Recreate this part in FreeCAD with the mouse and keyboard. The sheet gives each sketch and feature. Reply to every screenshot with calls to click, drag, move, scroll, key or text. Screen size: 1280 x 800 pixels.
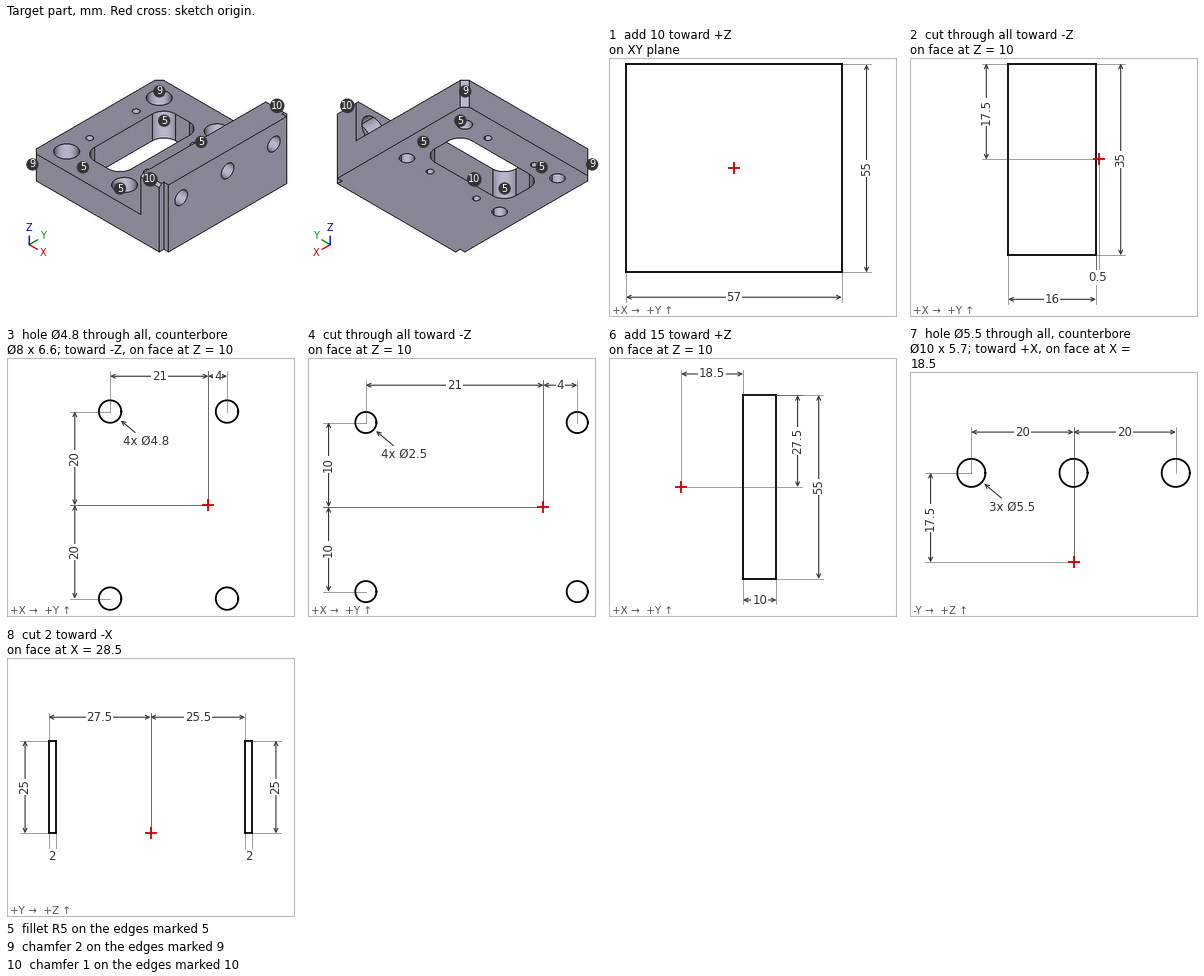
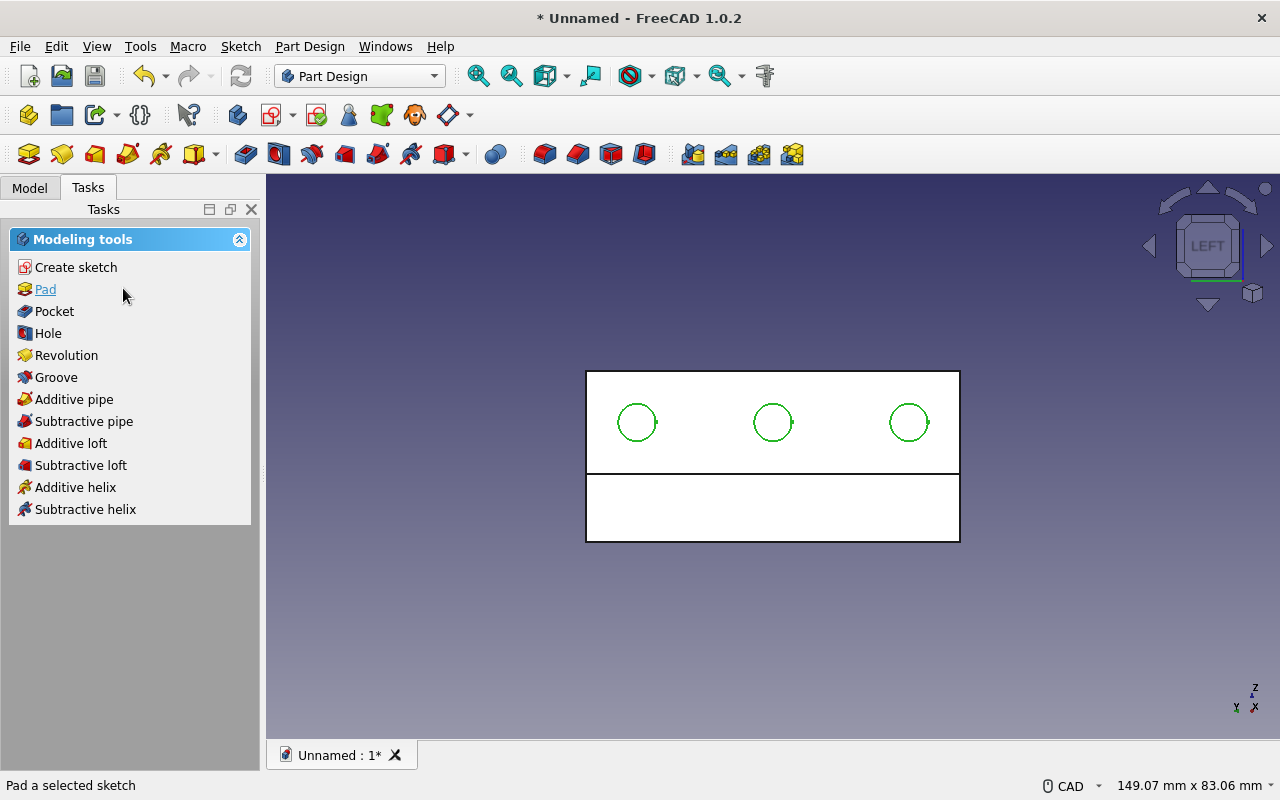
click(279, 154)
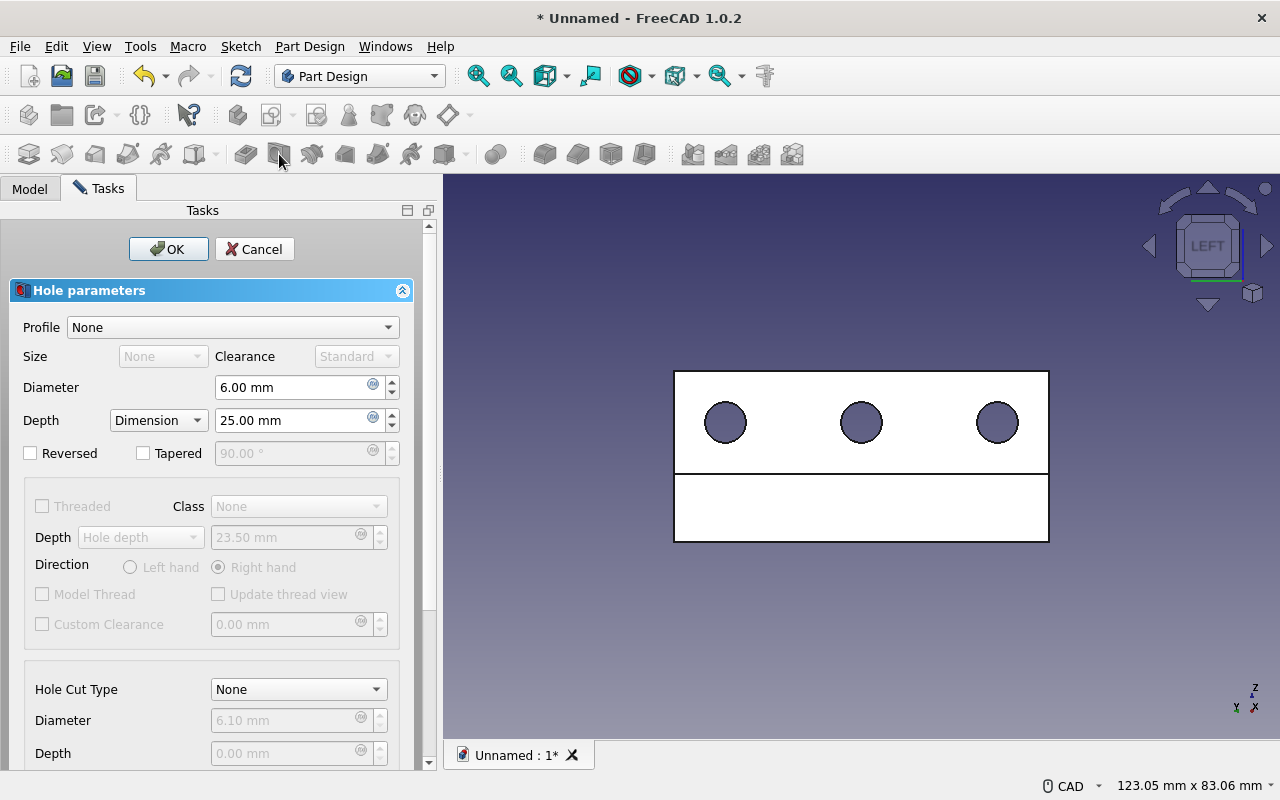
triple_click(300, 388)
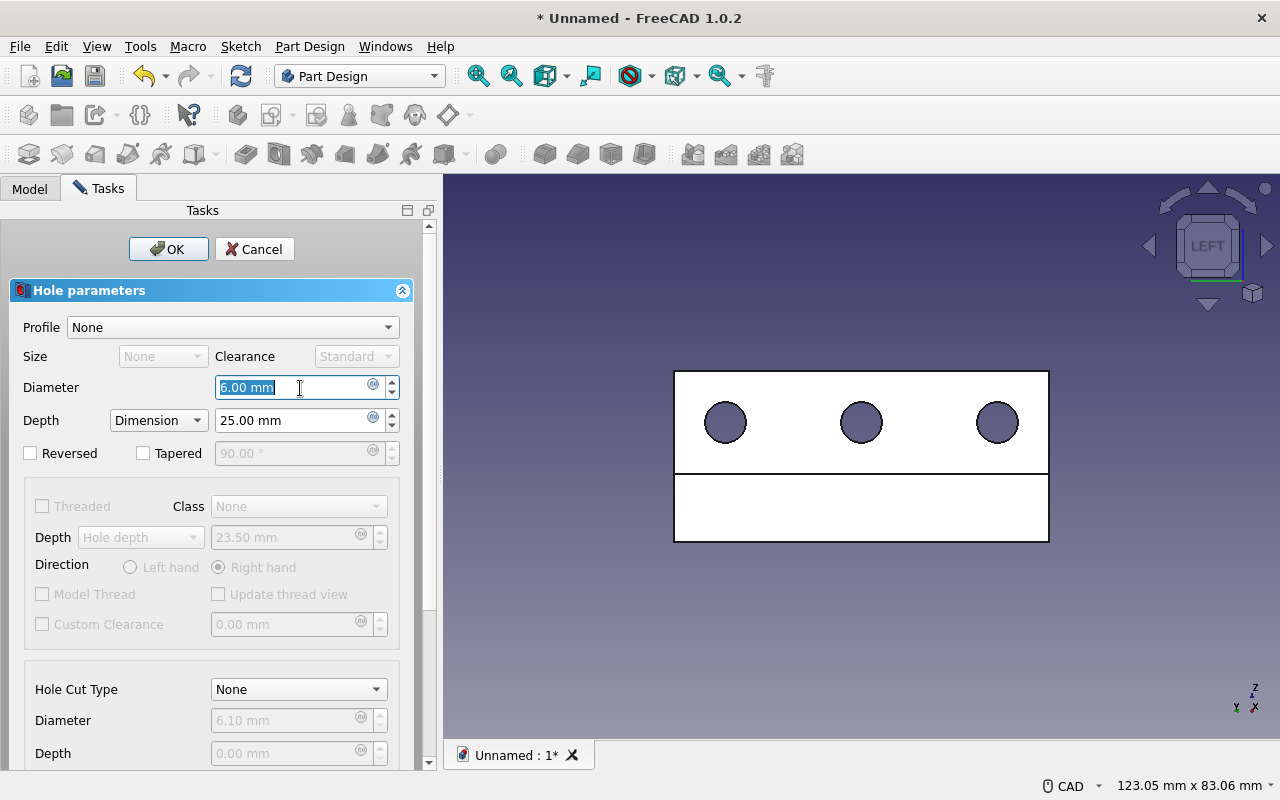
text(5.5)
key(Tab)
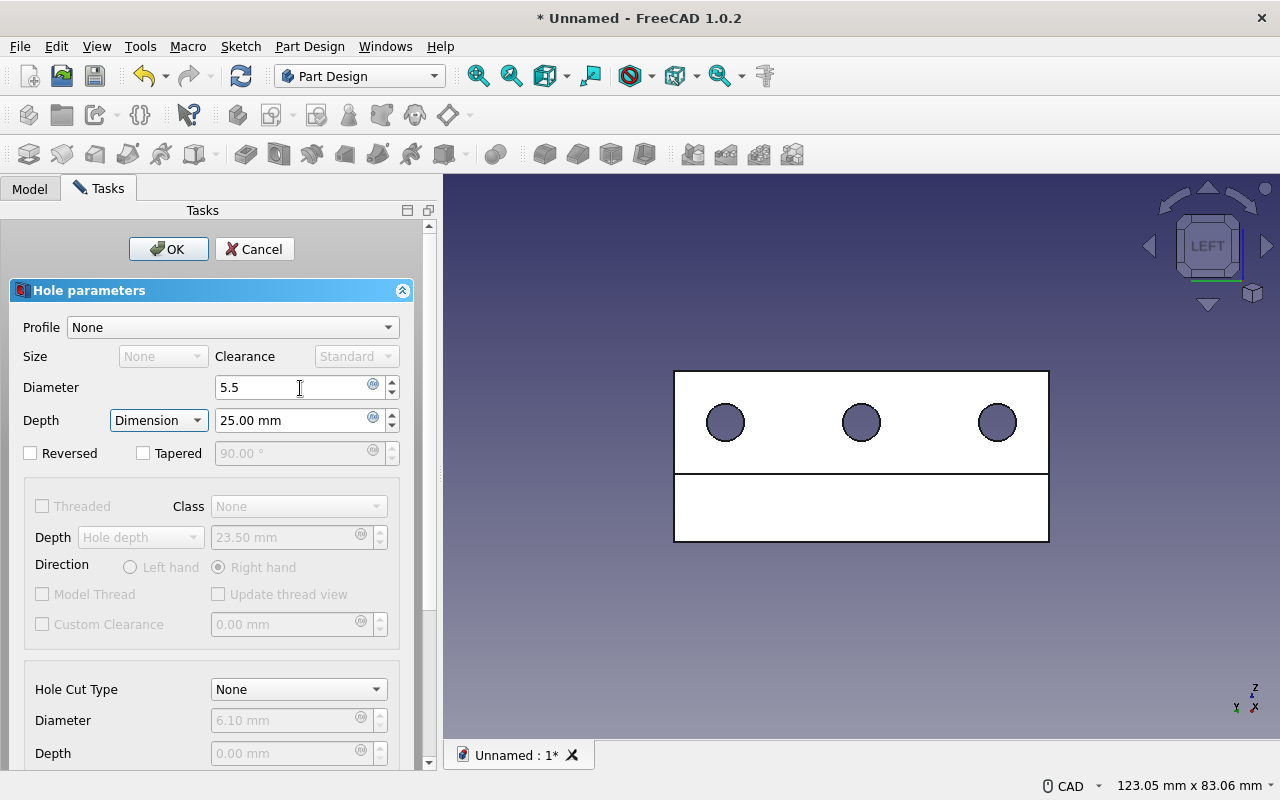
click(160, 420)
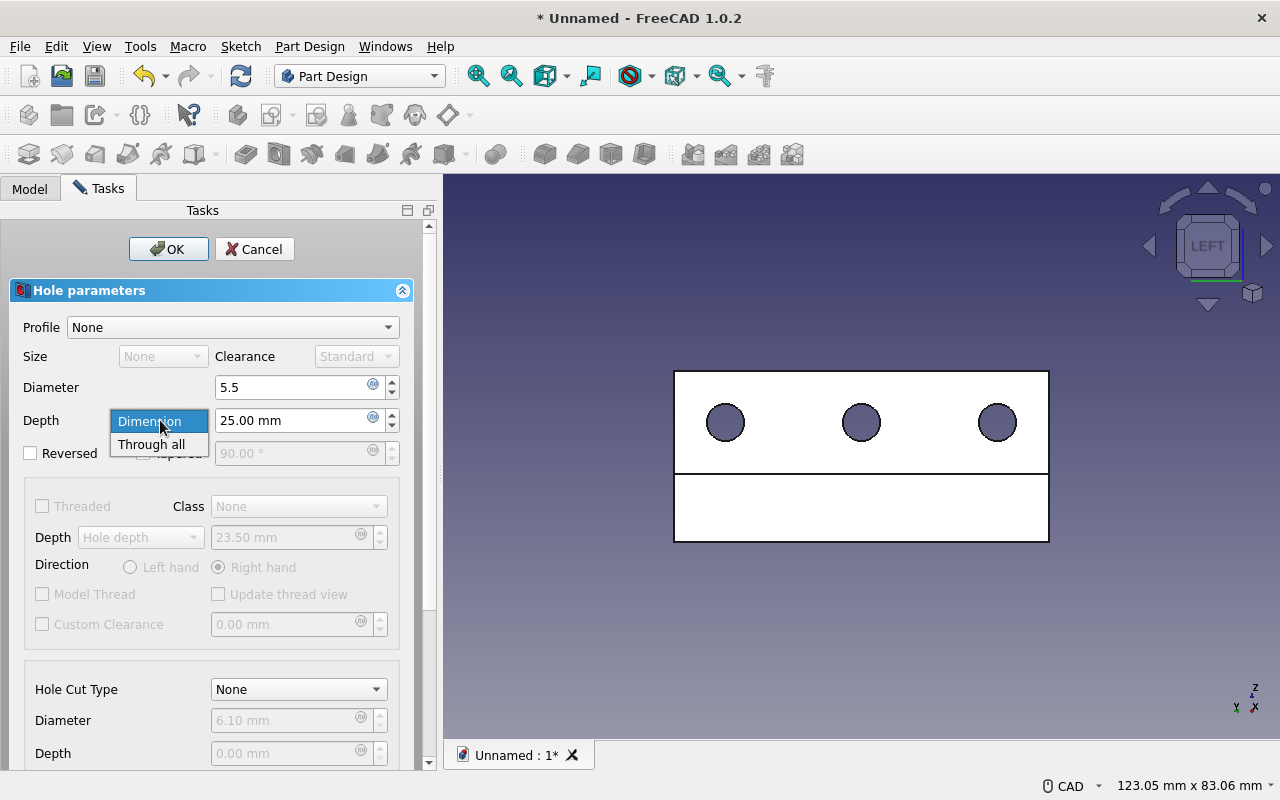
click(158, 444)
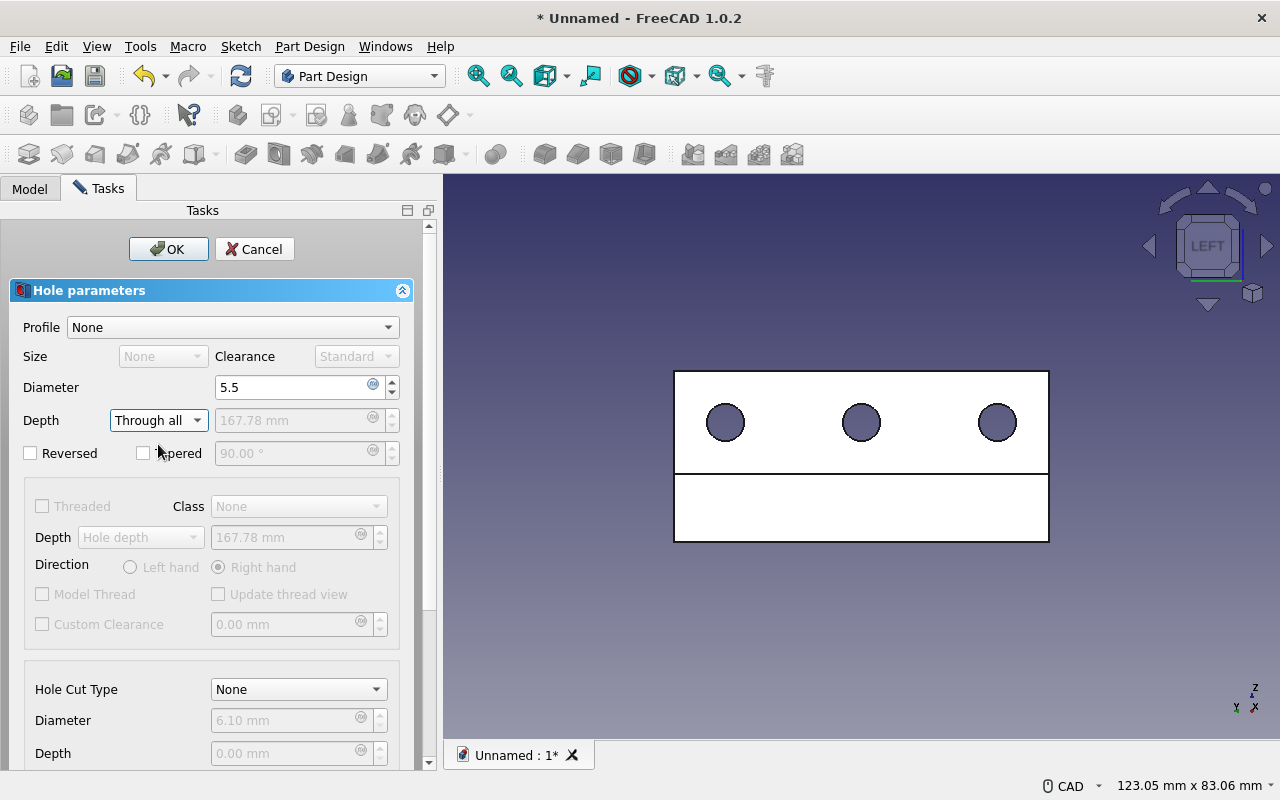
click(300, 690)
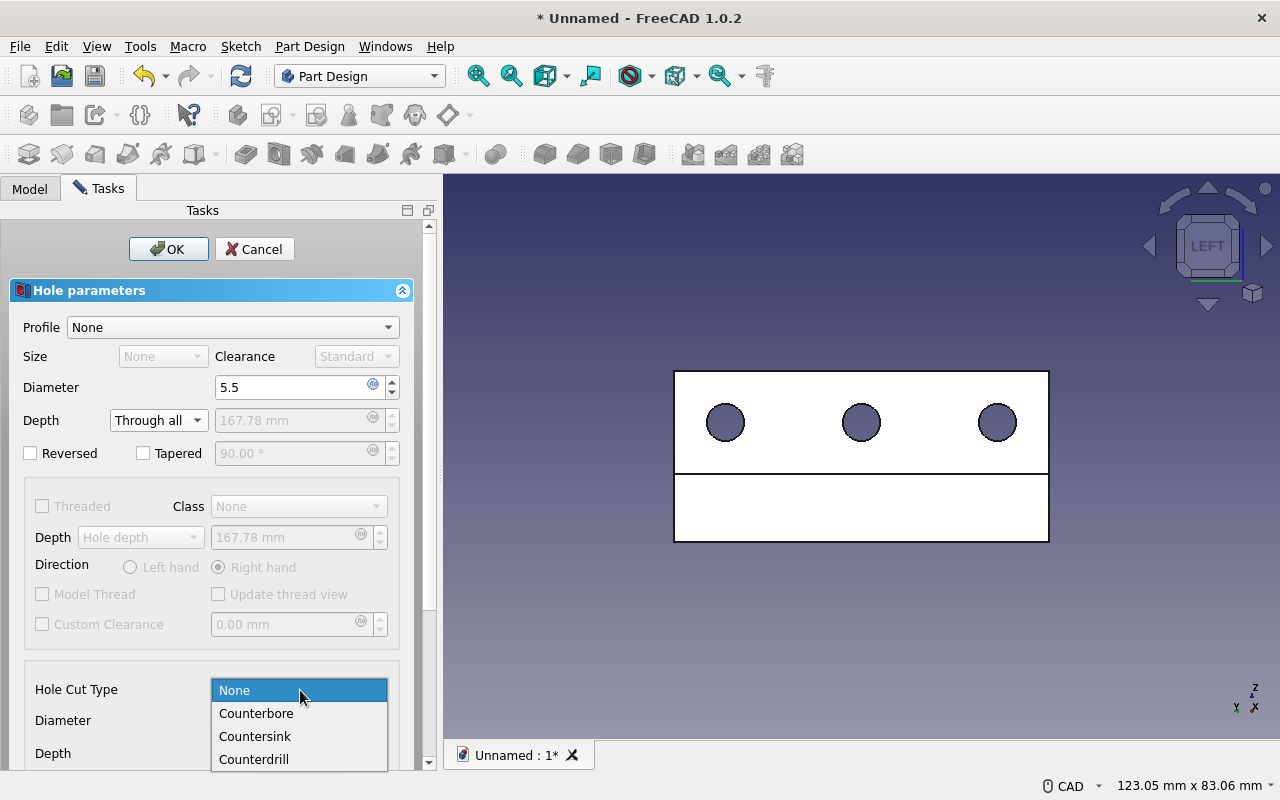
click(298, 714)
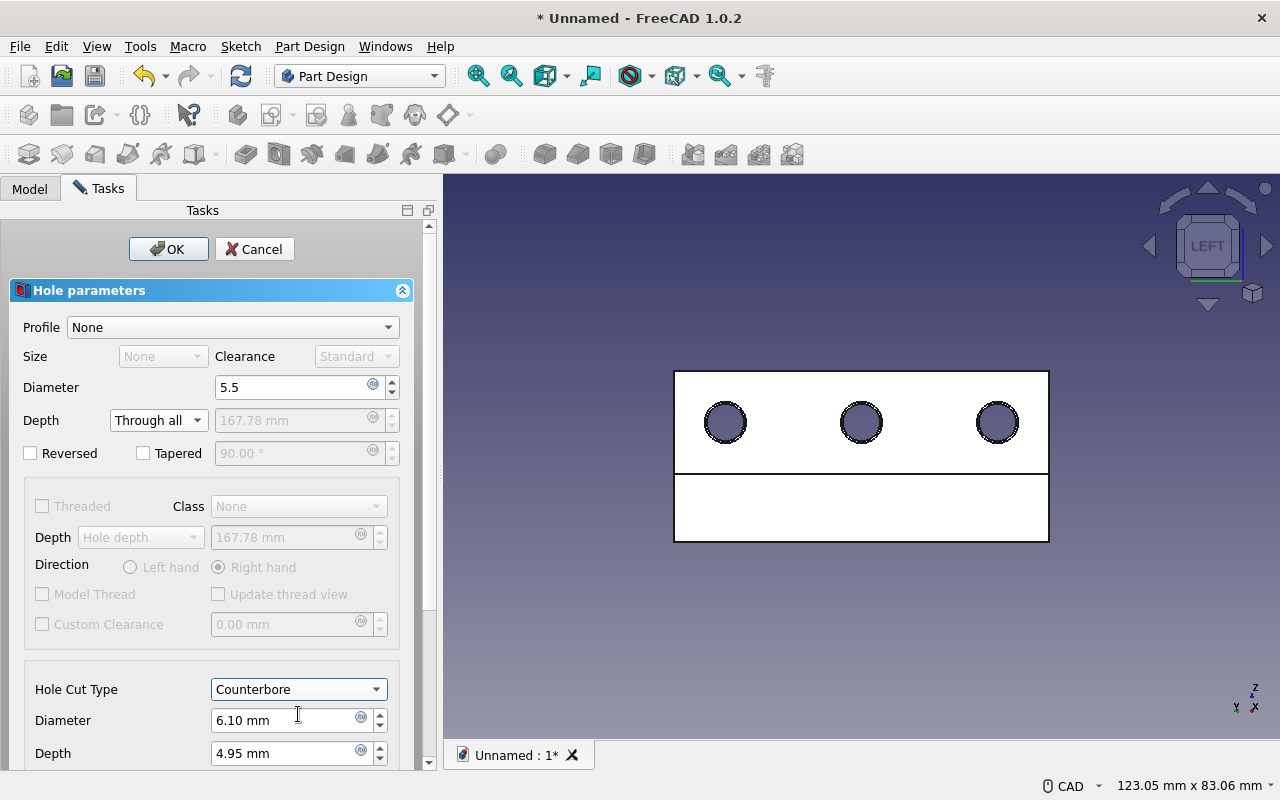
triple_click(292, 720)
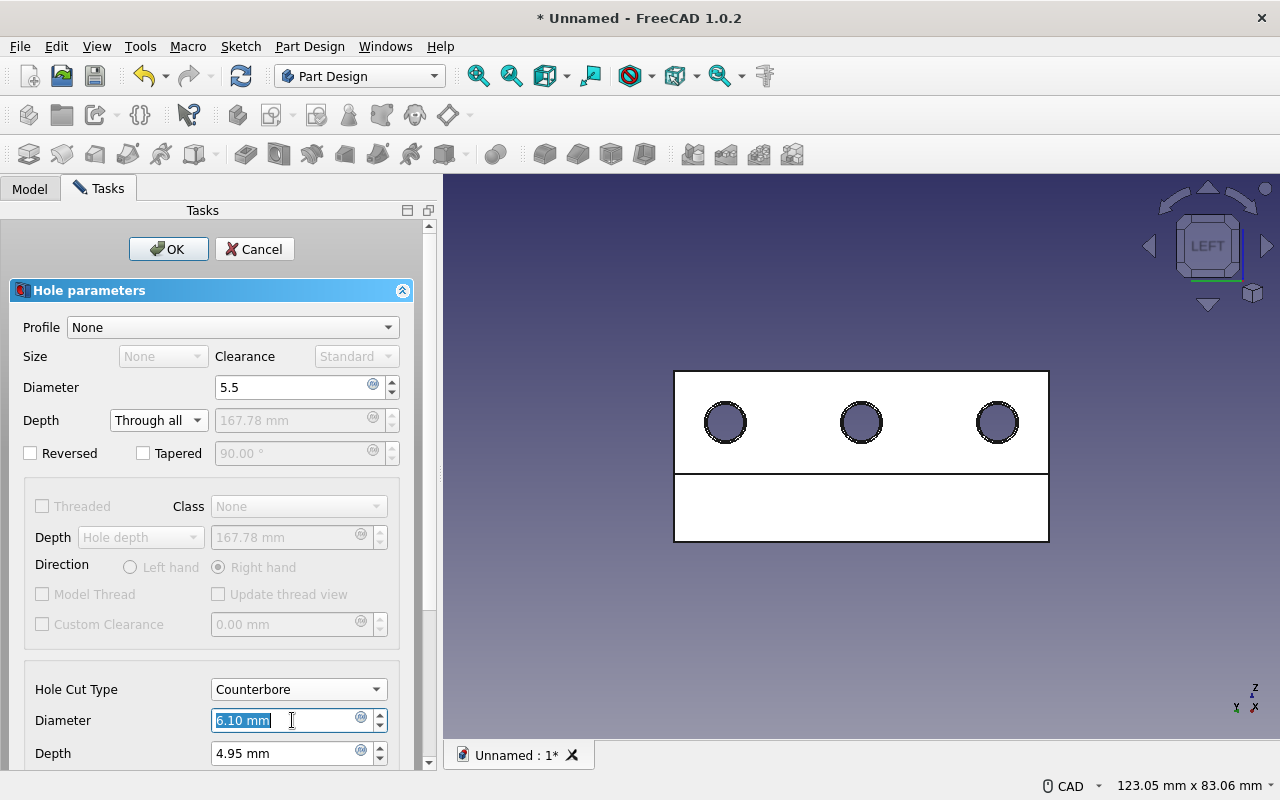
text(10)
key(Tab)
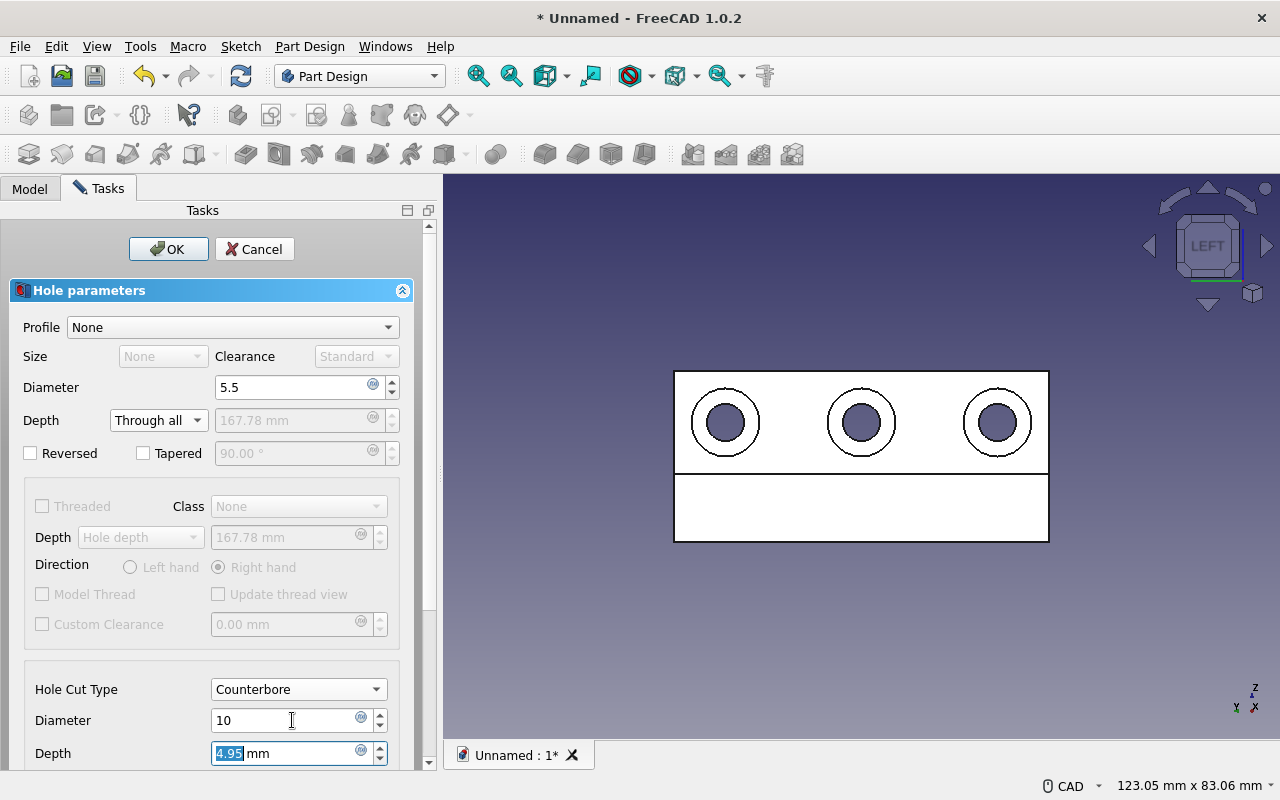
text(5.7)
key(Tab)